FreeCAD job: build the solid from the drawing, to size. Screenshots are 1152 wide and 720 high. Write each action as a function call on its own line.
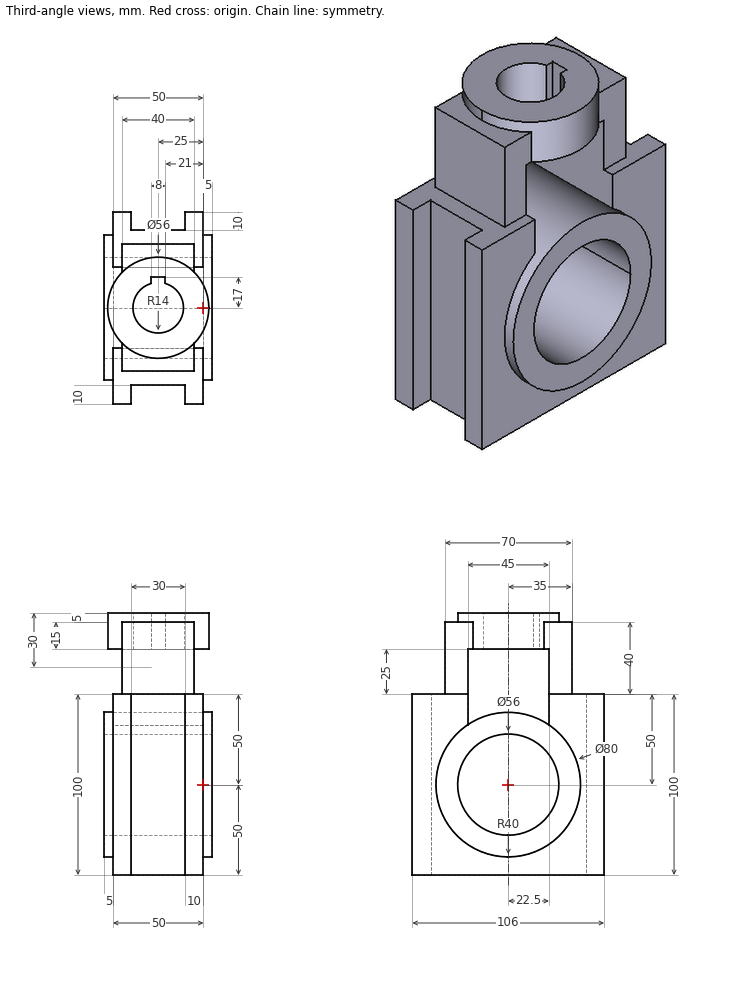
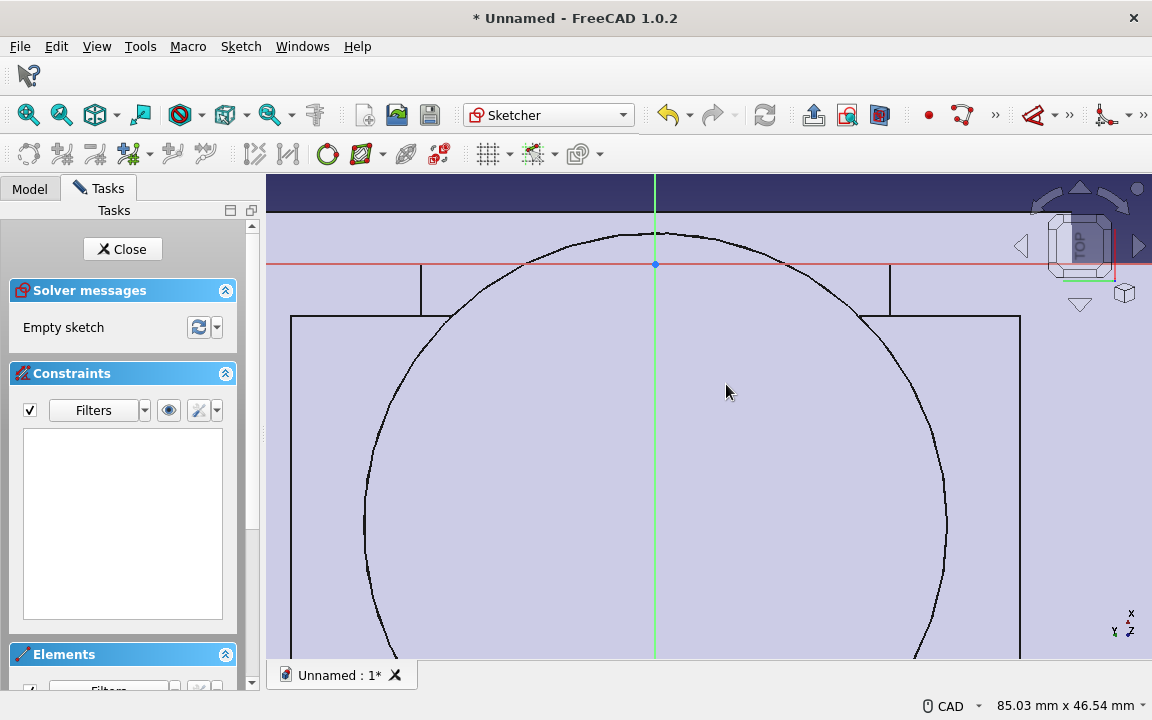
key(g)
key(m)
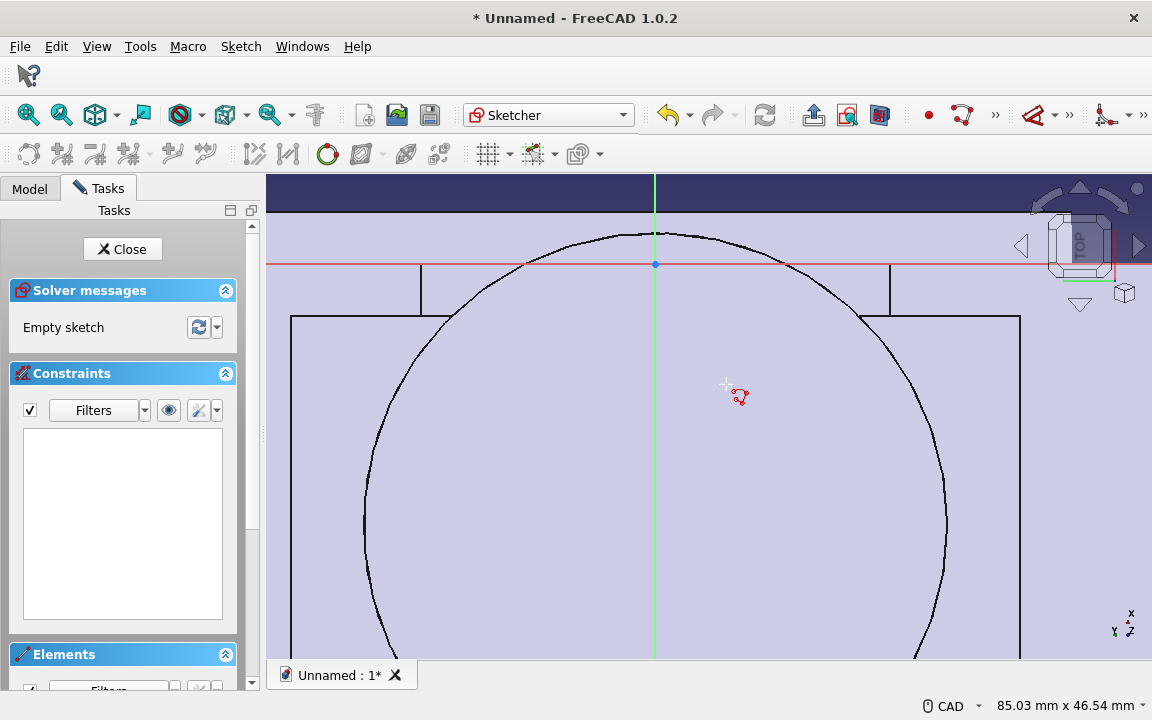
click(516, 483)
click(478, 483)
click(478, 567)
click(516, 567)
right_click(516, 567)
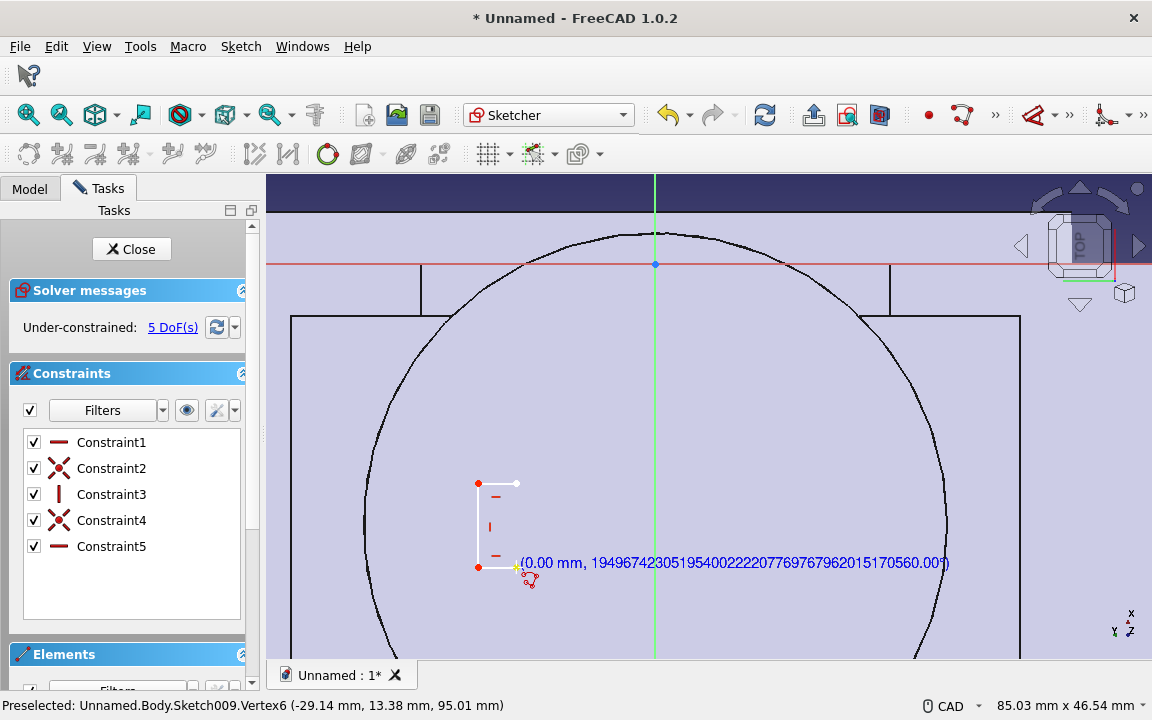
key(g)
key(3)
key(a)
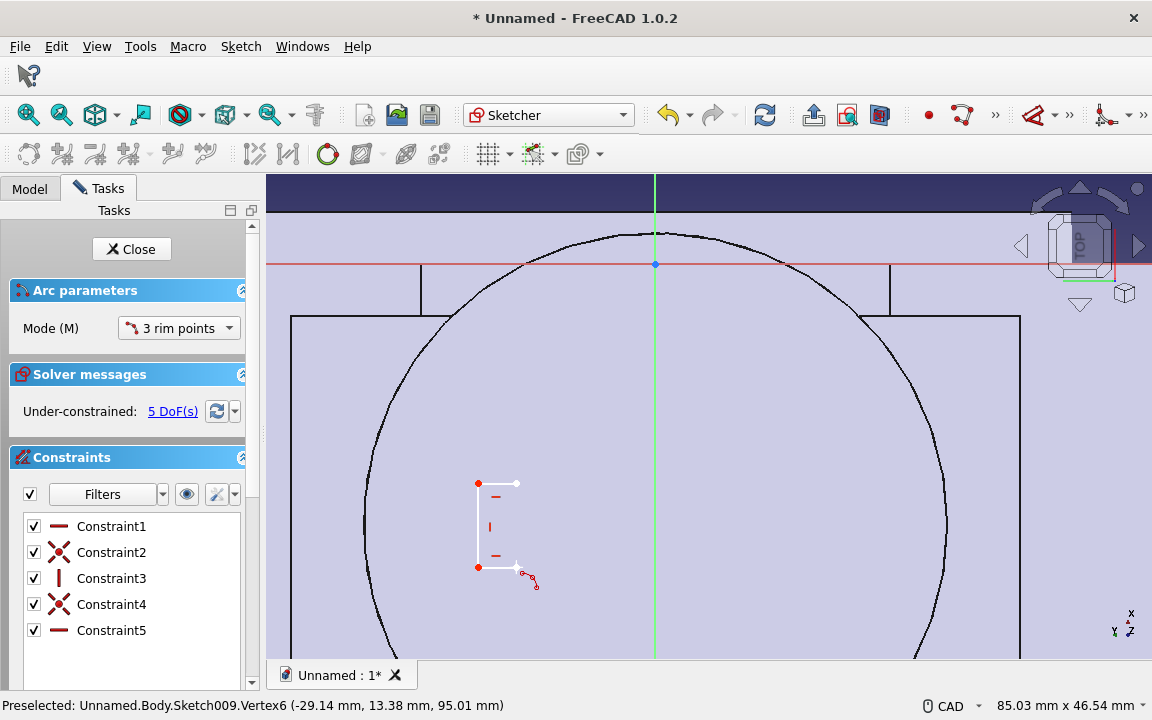
click(516, 568)
click(516, 484)
click(801, 525)
key(Escape)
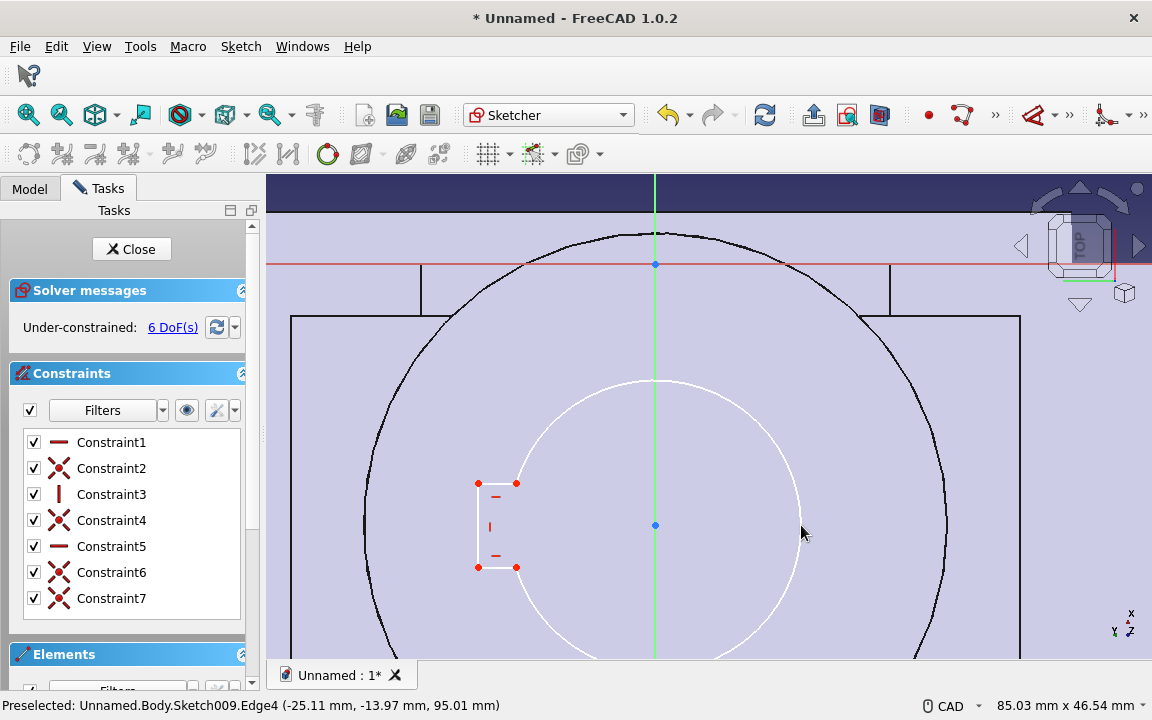
click(655, 526)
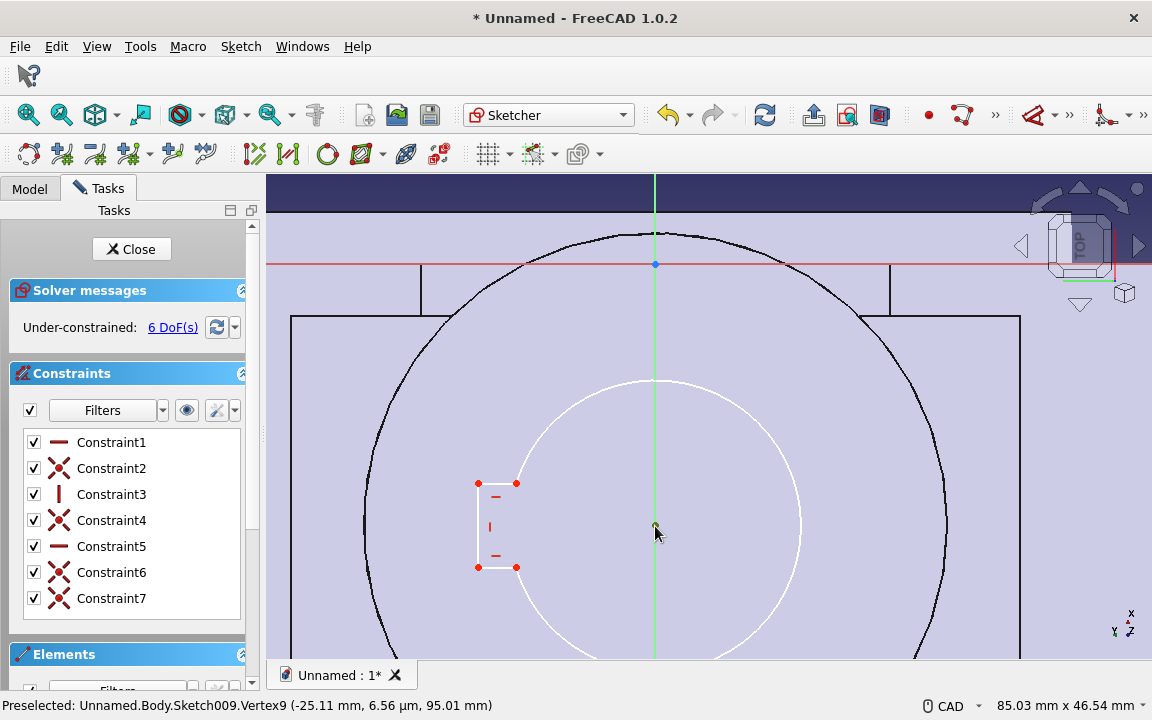
click(655, 600)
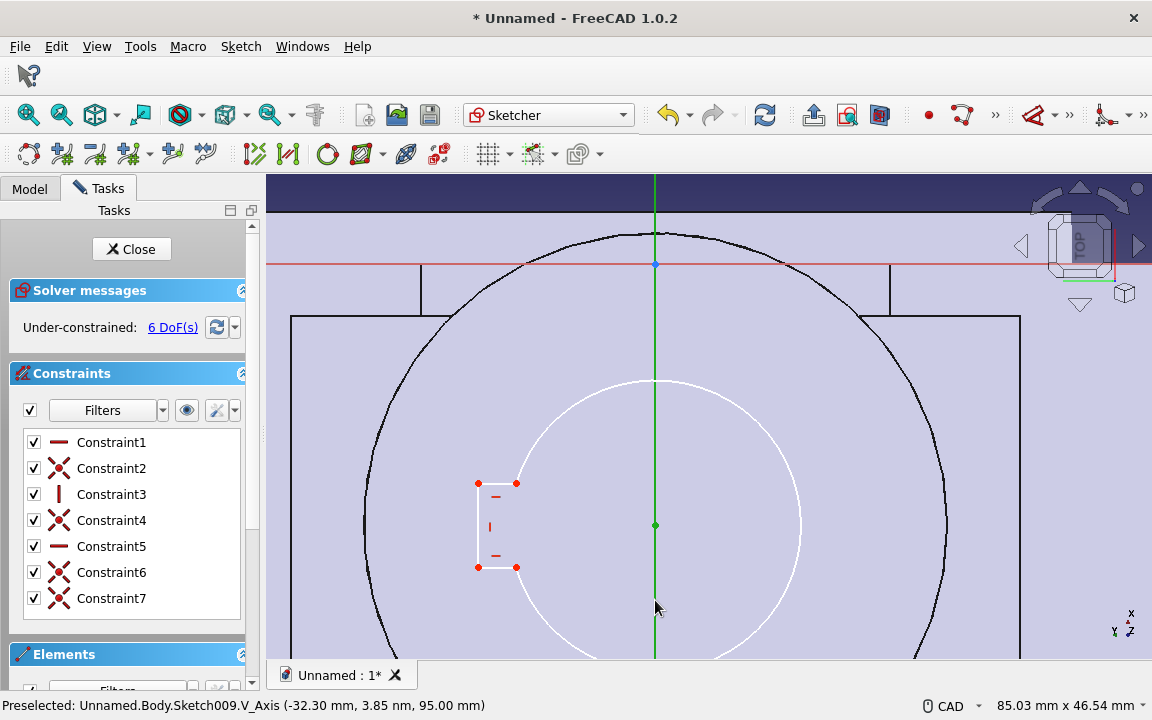
key(c)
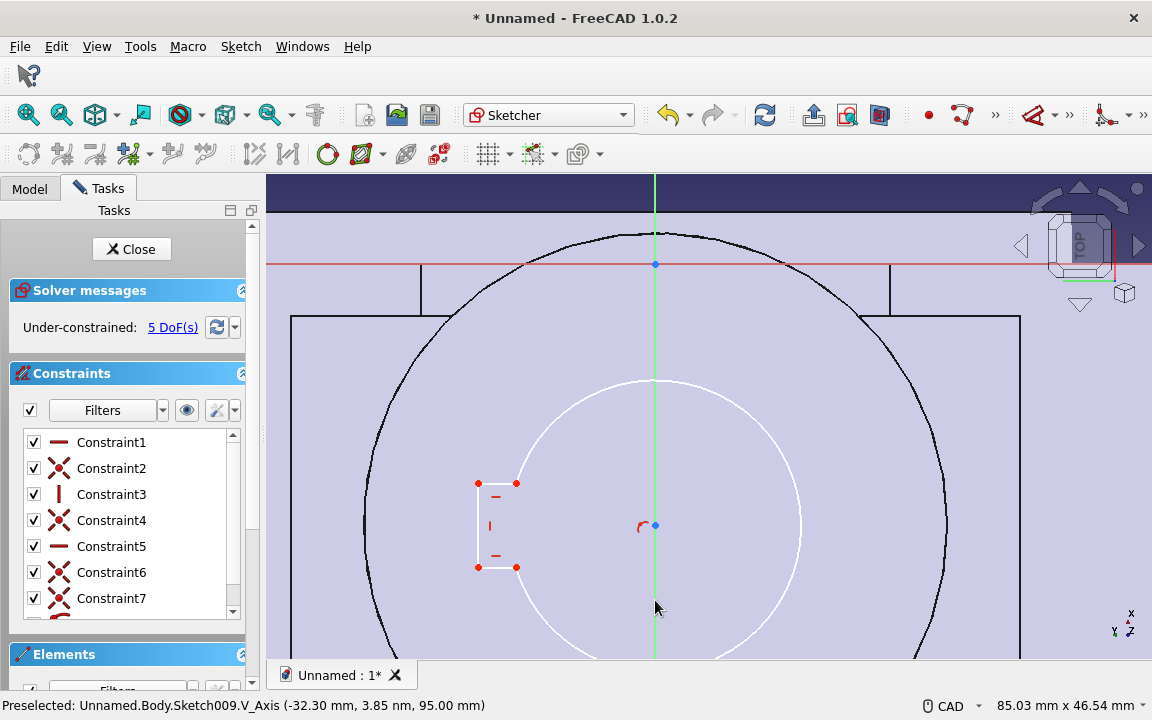
click(1032, 116)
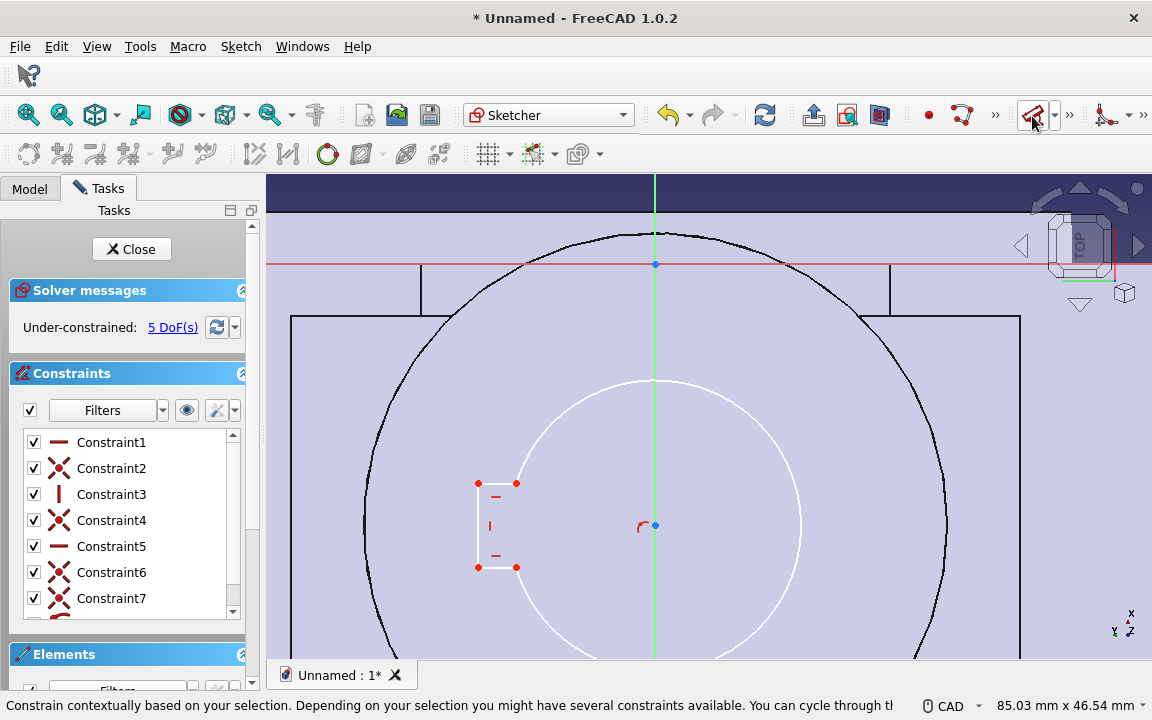
click(716, 394)
click(729, 365)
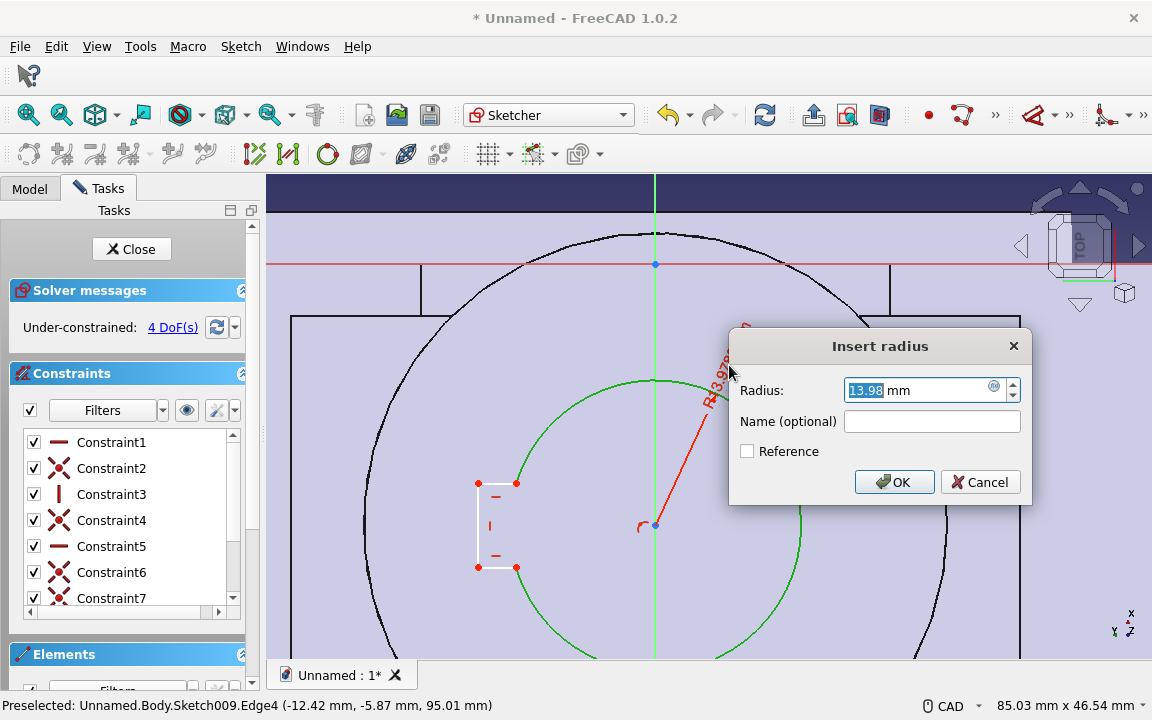
text(14)
key(Return)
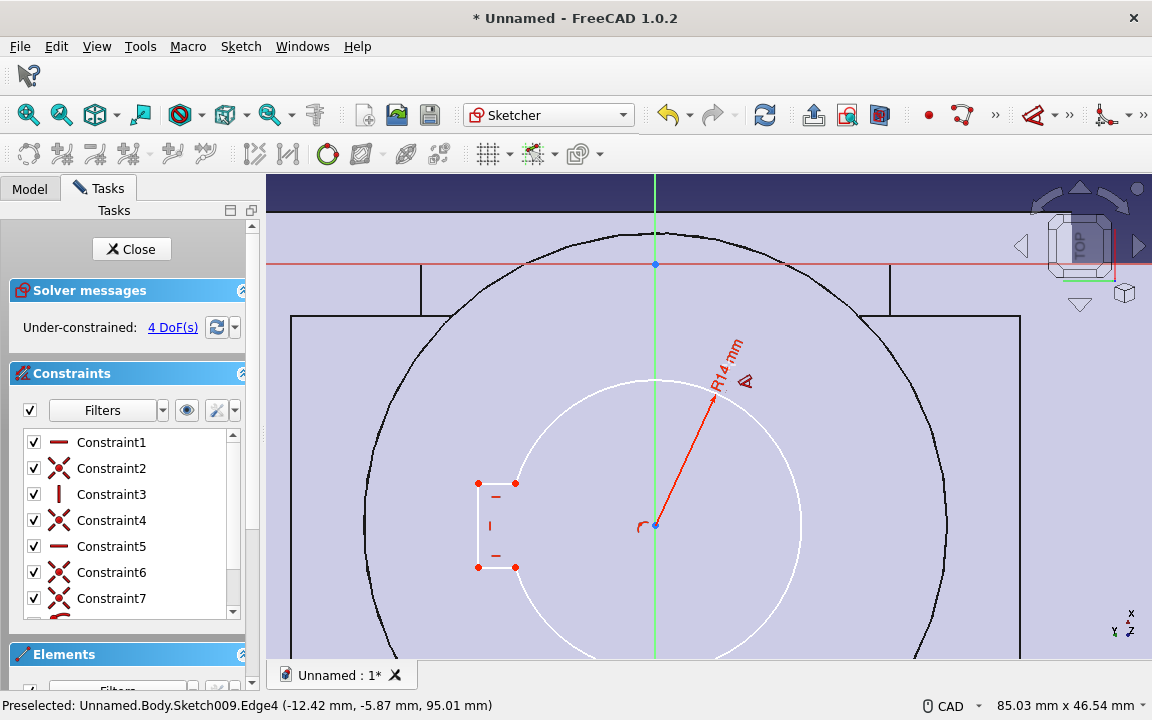
click(478, 509)
click(444, 526)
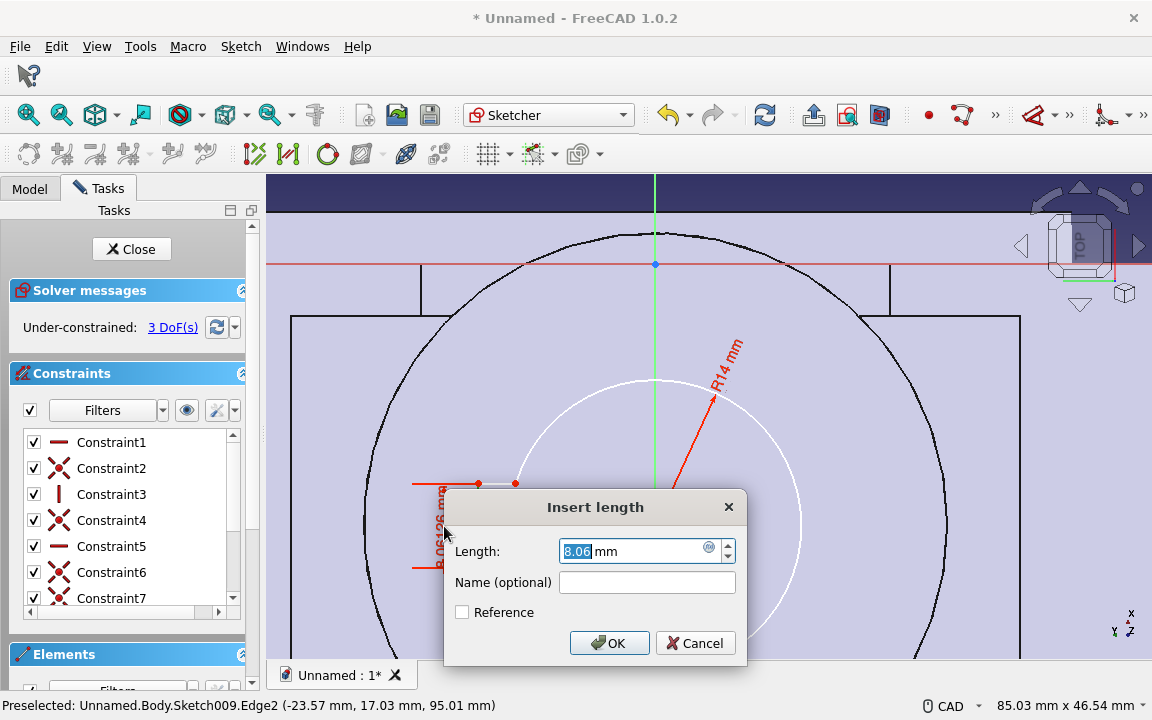
text(8)
key(Return)